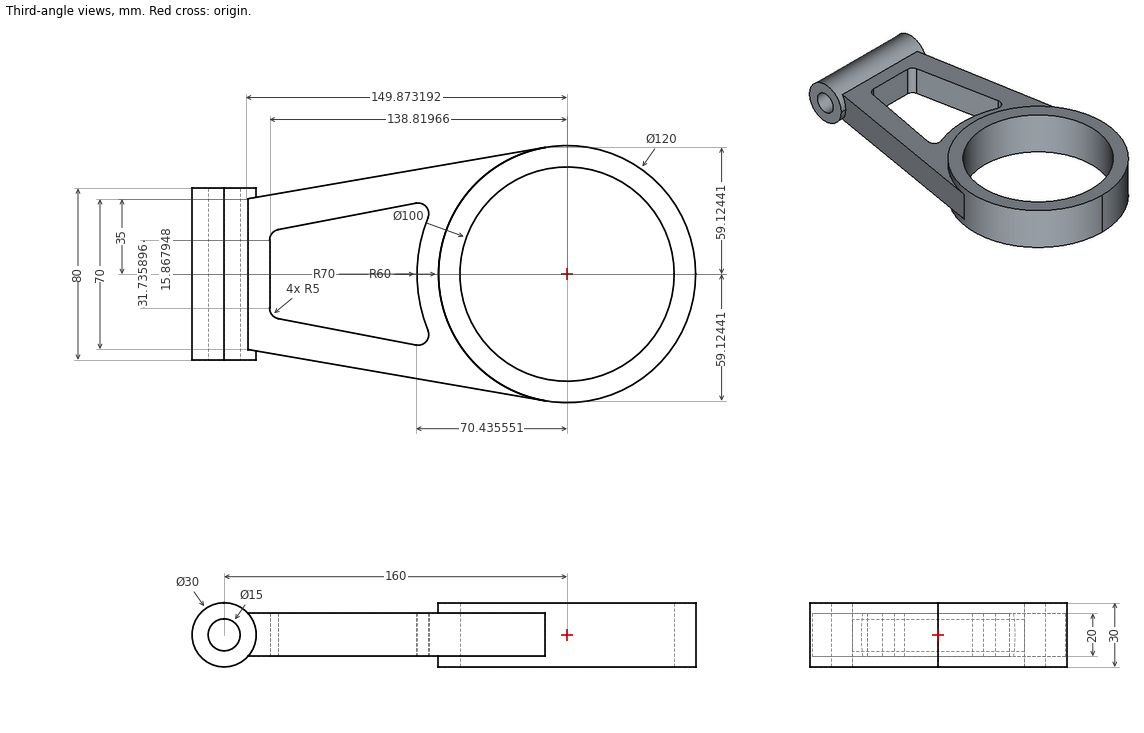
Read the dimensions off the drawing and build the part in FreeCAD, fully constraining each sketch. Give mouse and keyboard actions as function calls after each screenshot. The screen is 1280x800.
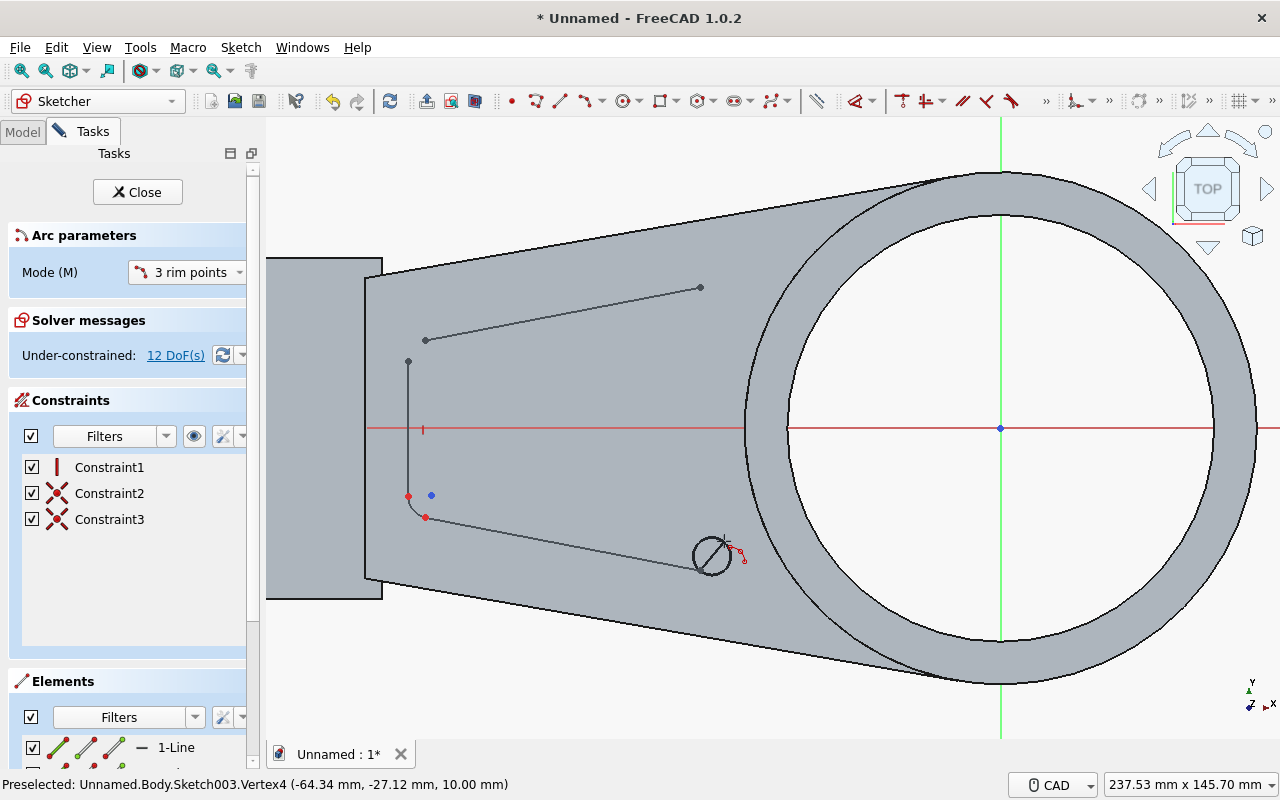
scroll(721, 562, up, 2)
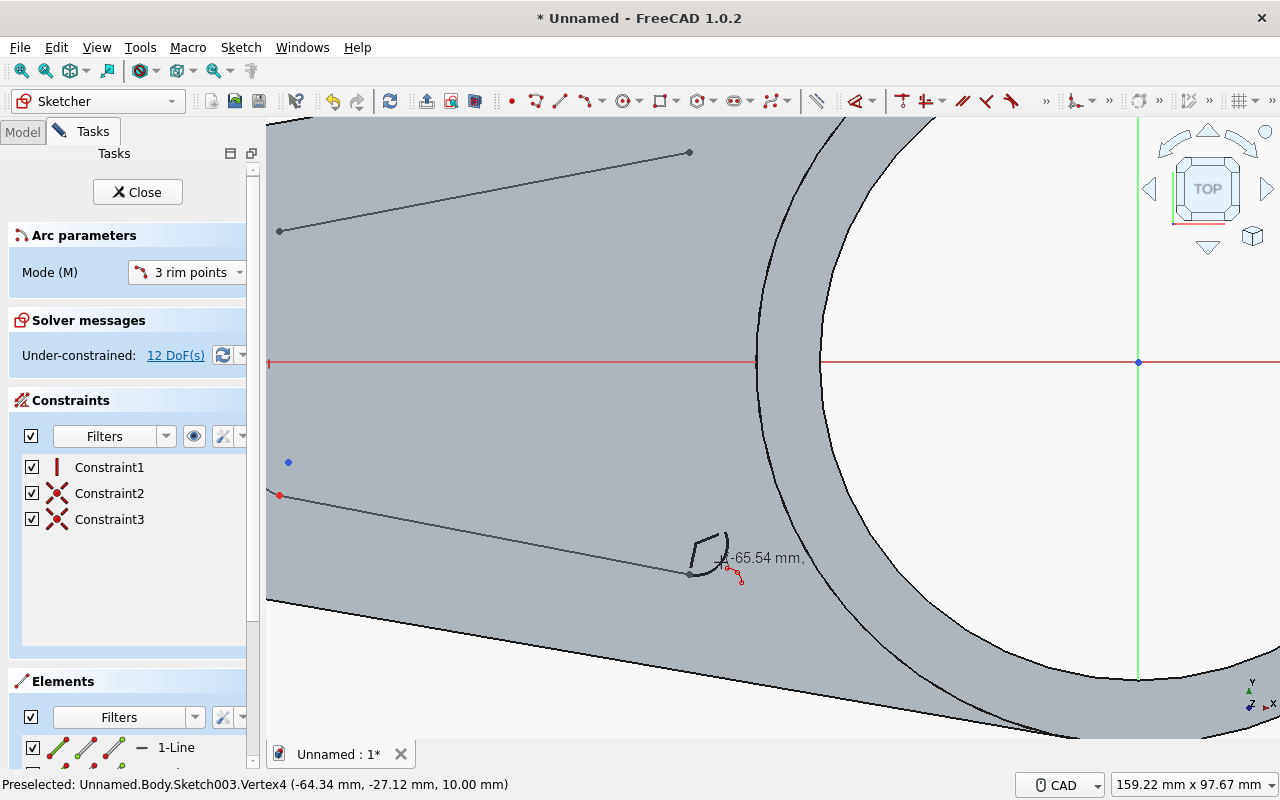
click(720, 562)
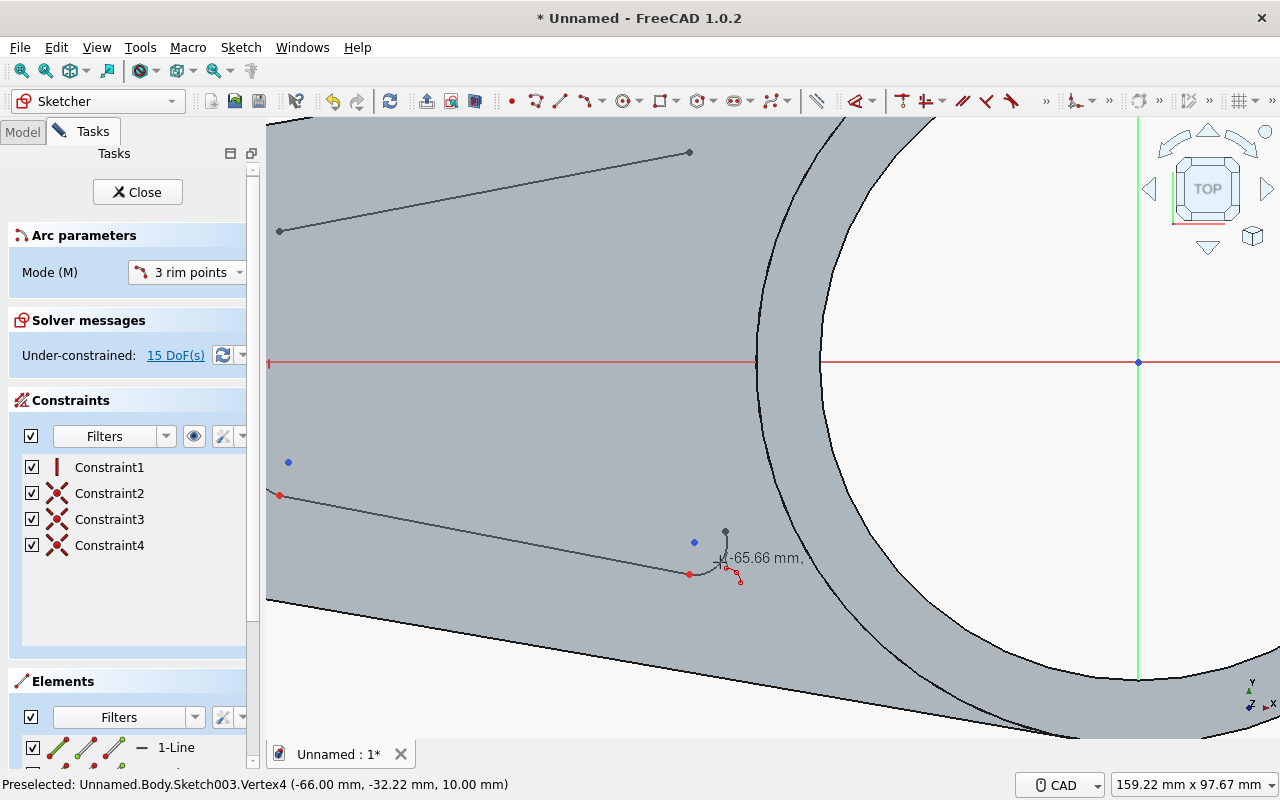
click(725, 532)
click(725, 195)
click(694, 328)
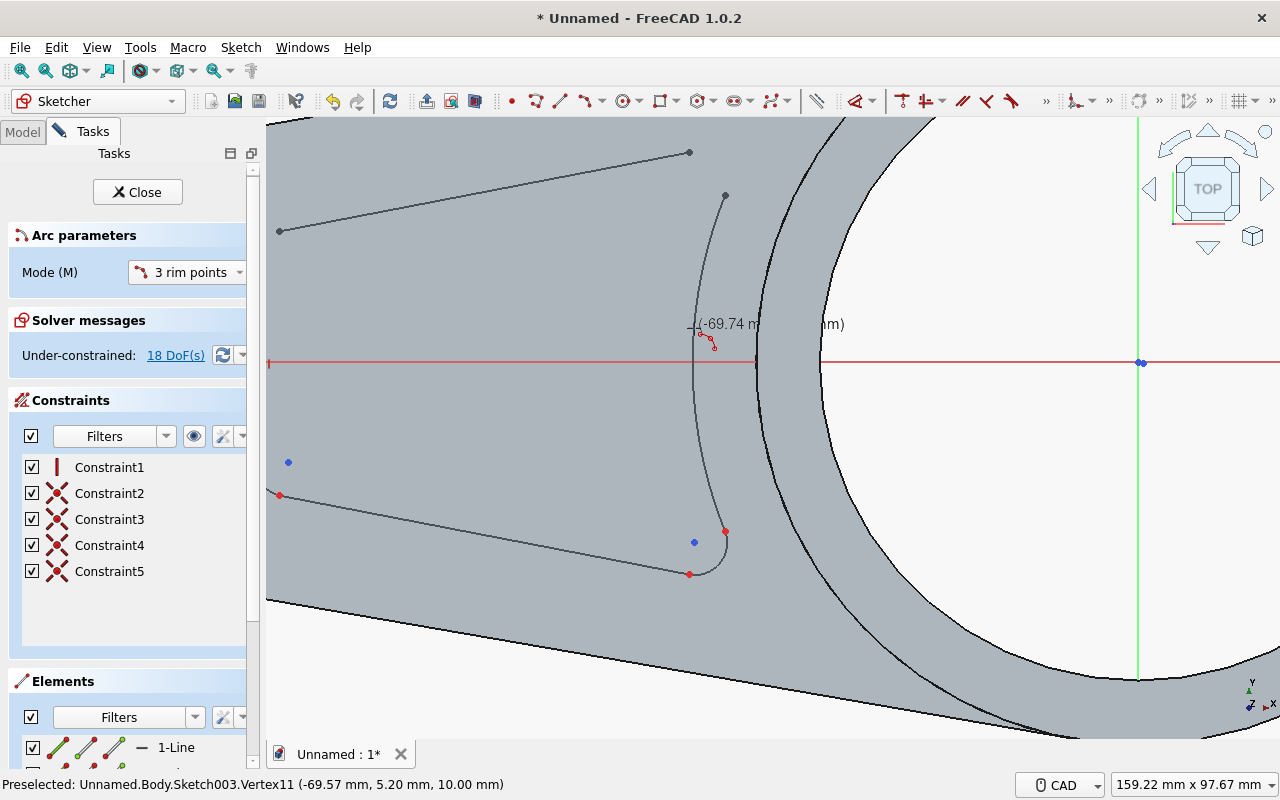
click(725, 196)
click(689, 152)
click(720, 162)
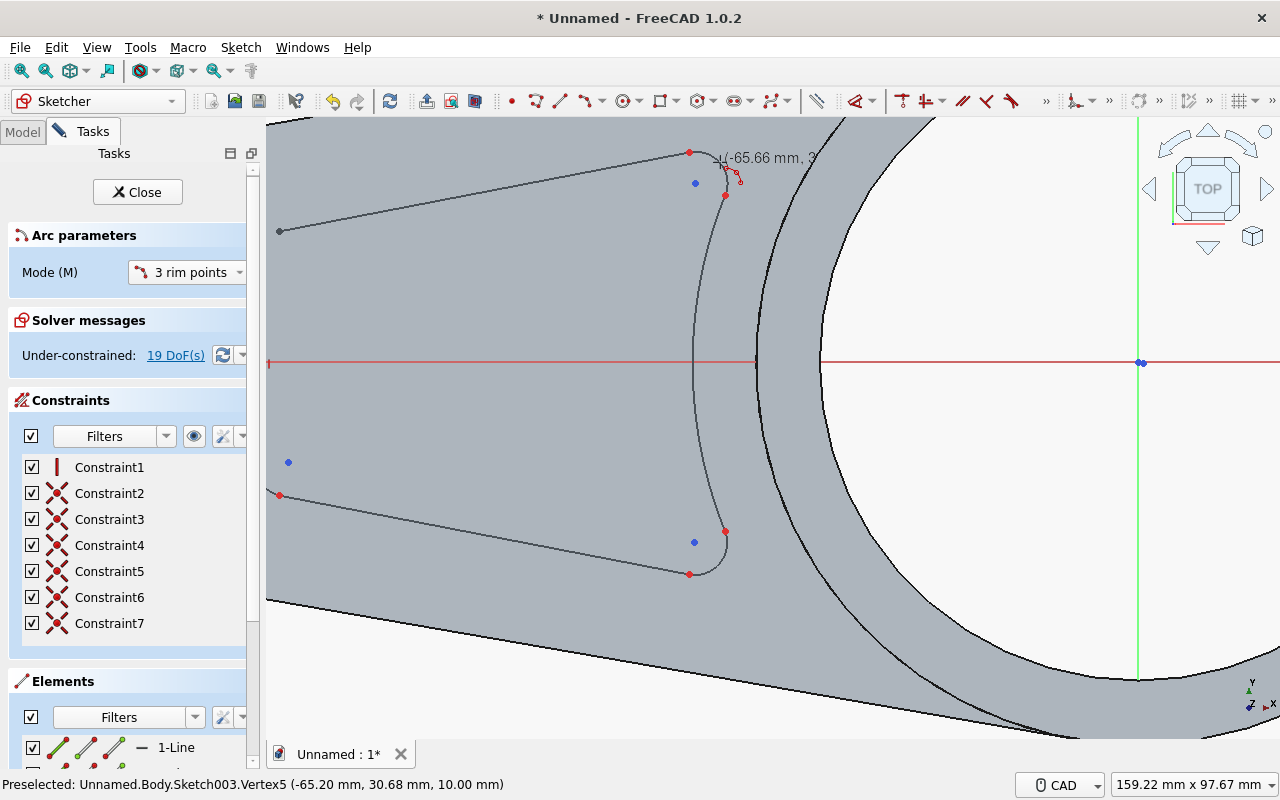
scroll(722, 562, down, 2)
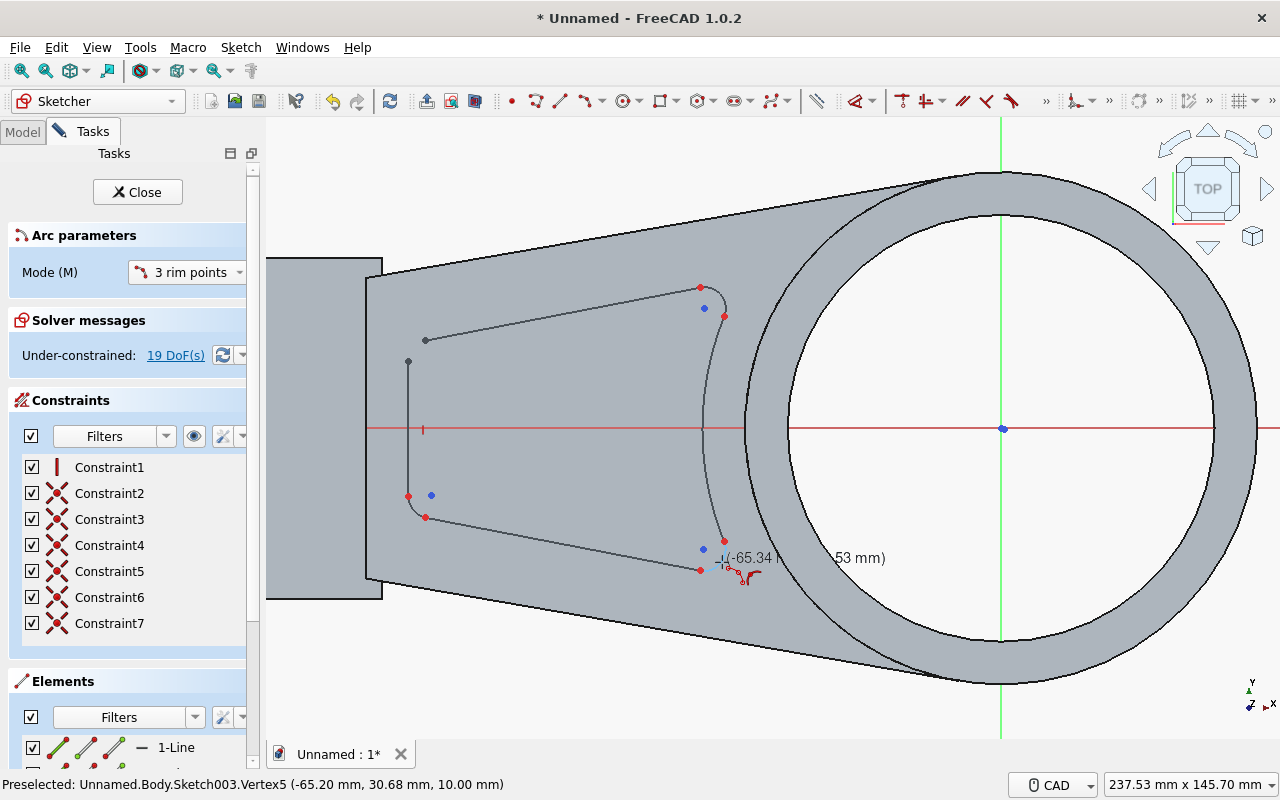
click(425, 341)
click(408, 362)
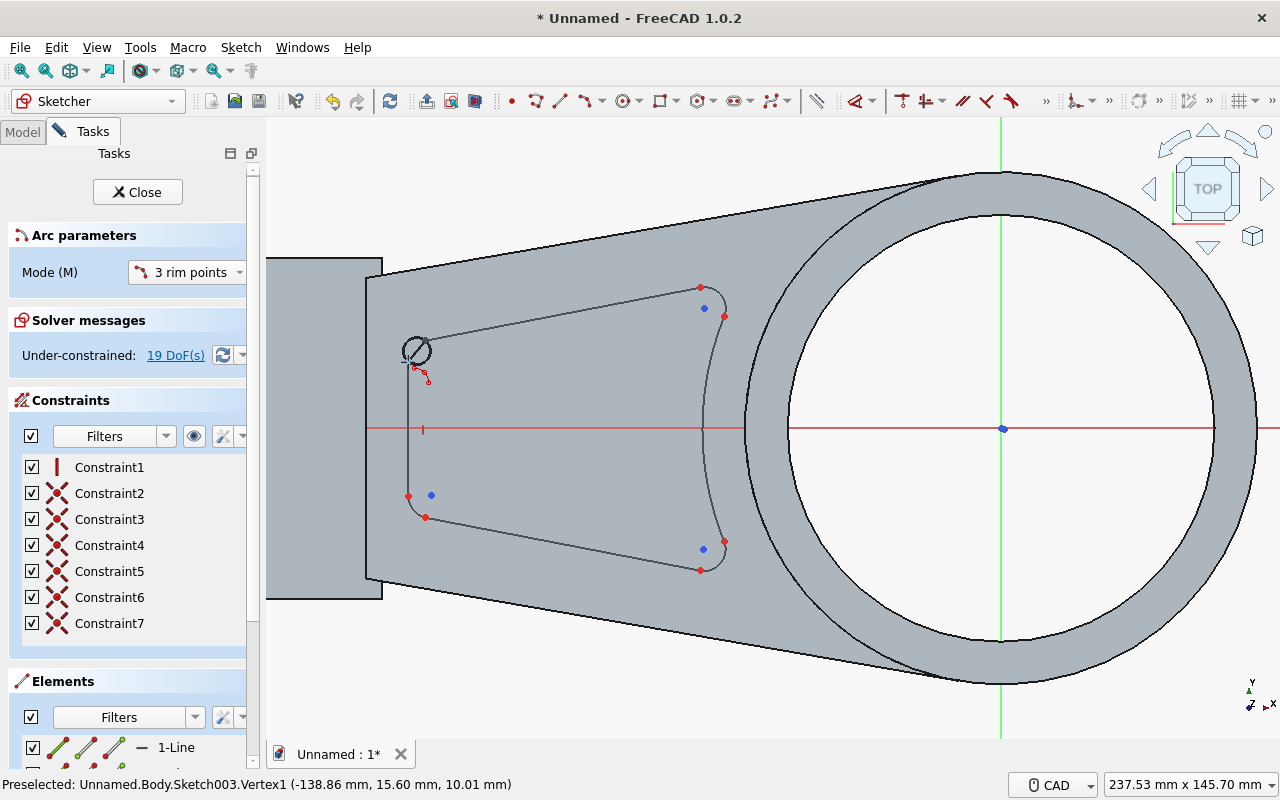
scroll(413, 347, up, 6)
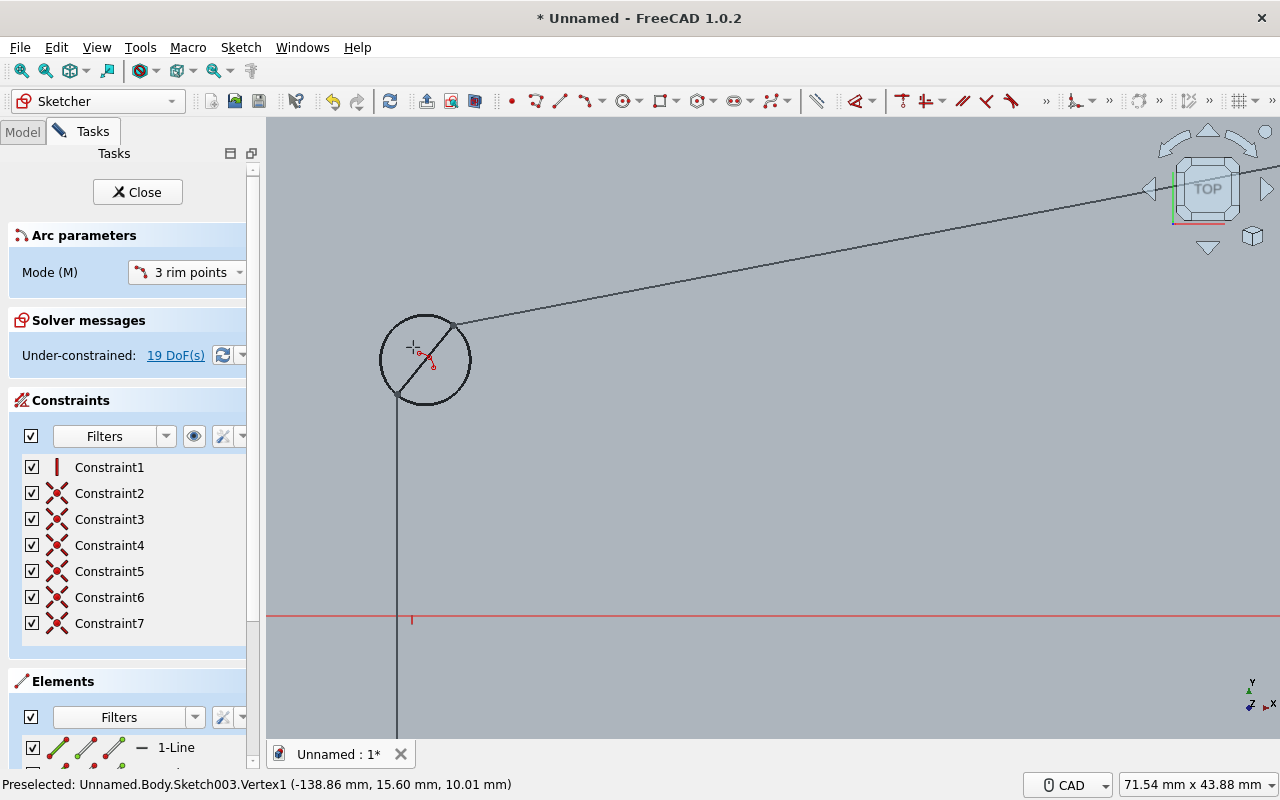
click(414, 346)
key(Escape)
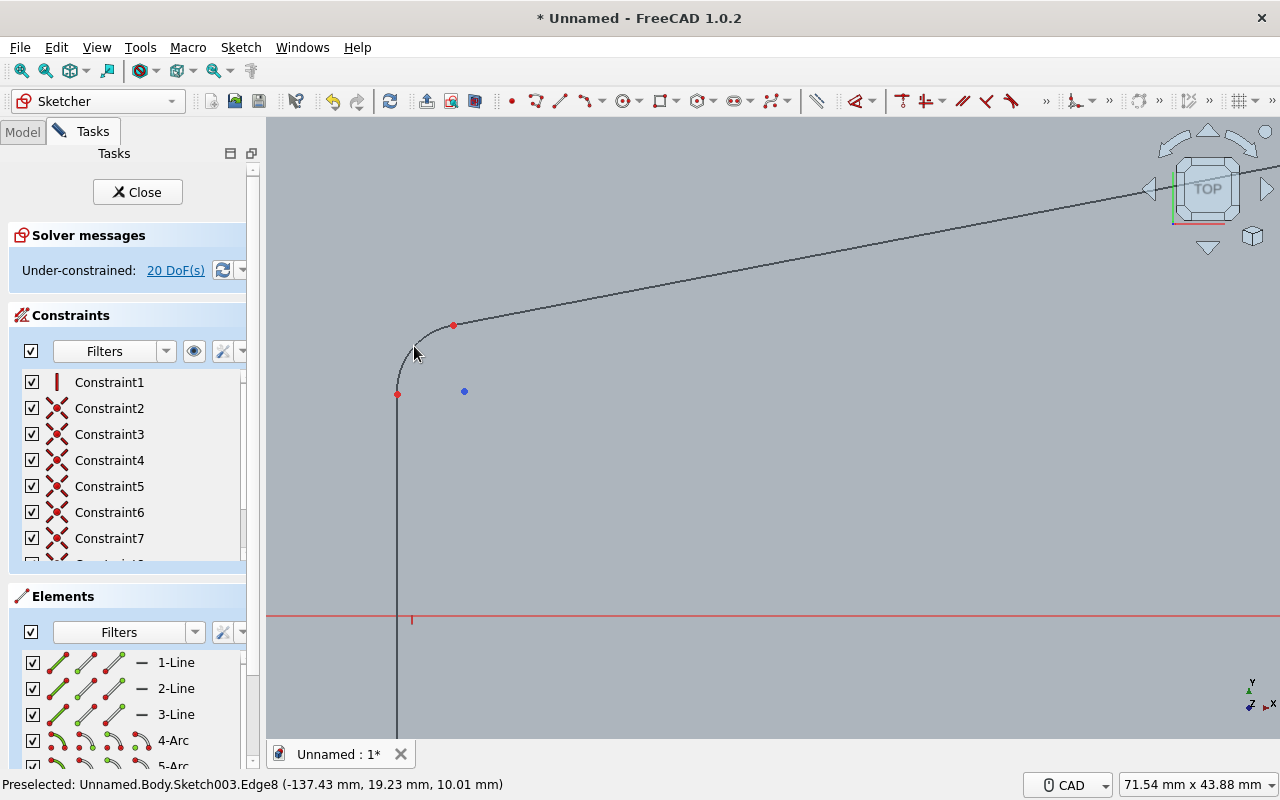
click(397, 529)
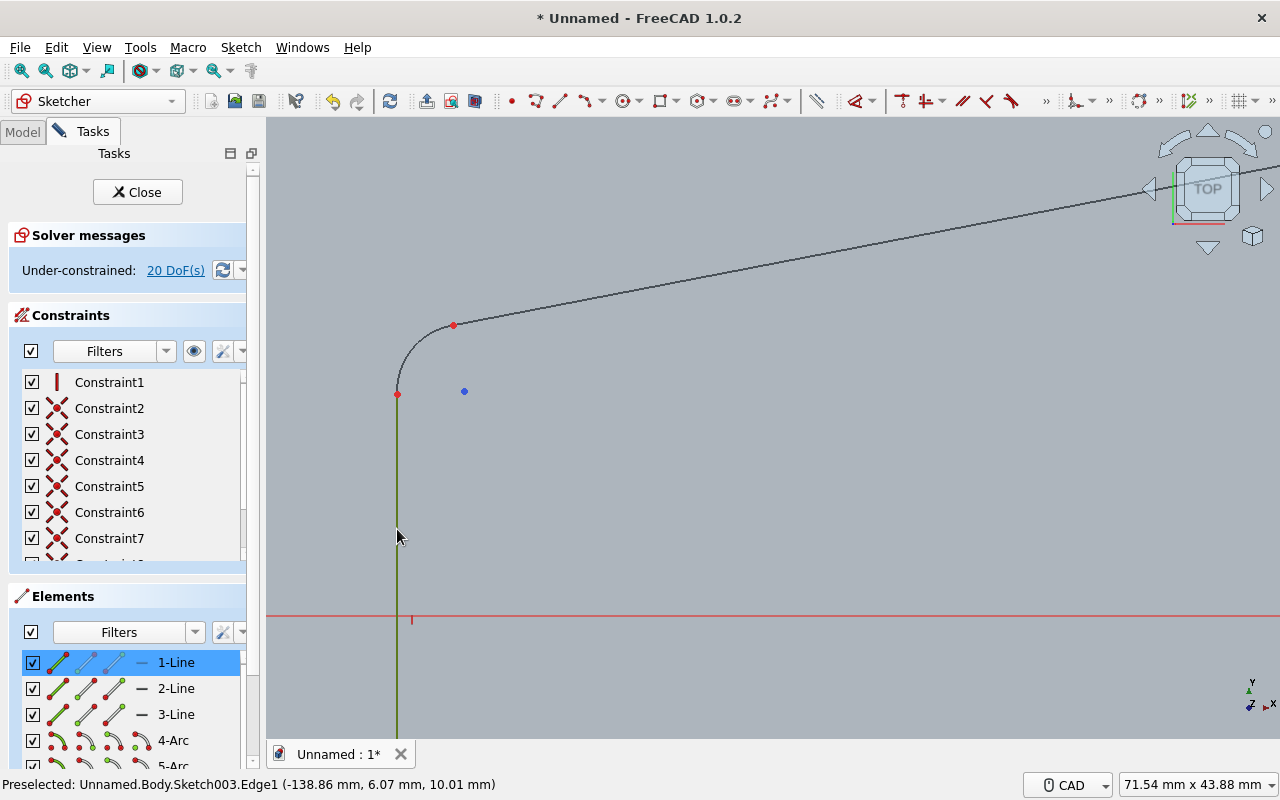
scroll(413, 347, down, 6)